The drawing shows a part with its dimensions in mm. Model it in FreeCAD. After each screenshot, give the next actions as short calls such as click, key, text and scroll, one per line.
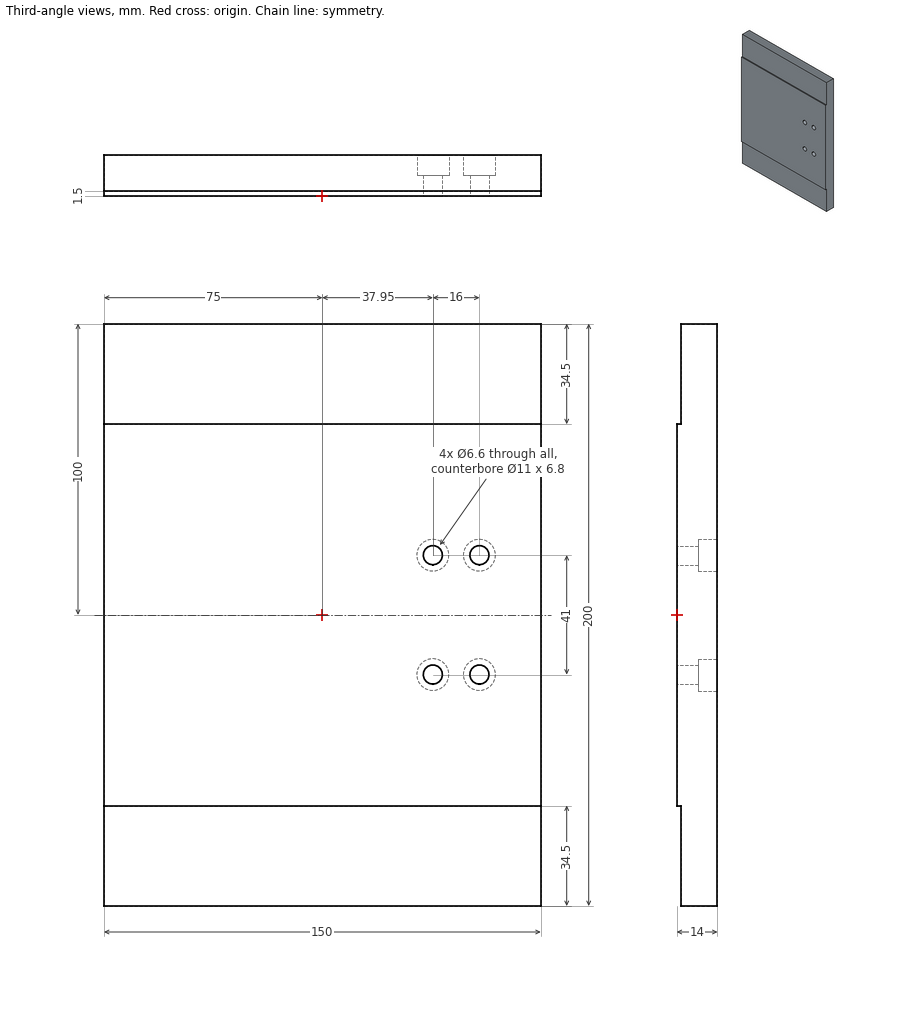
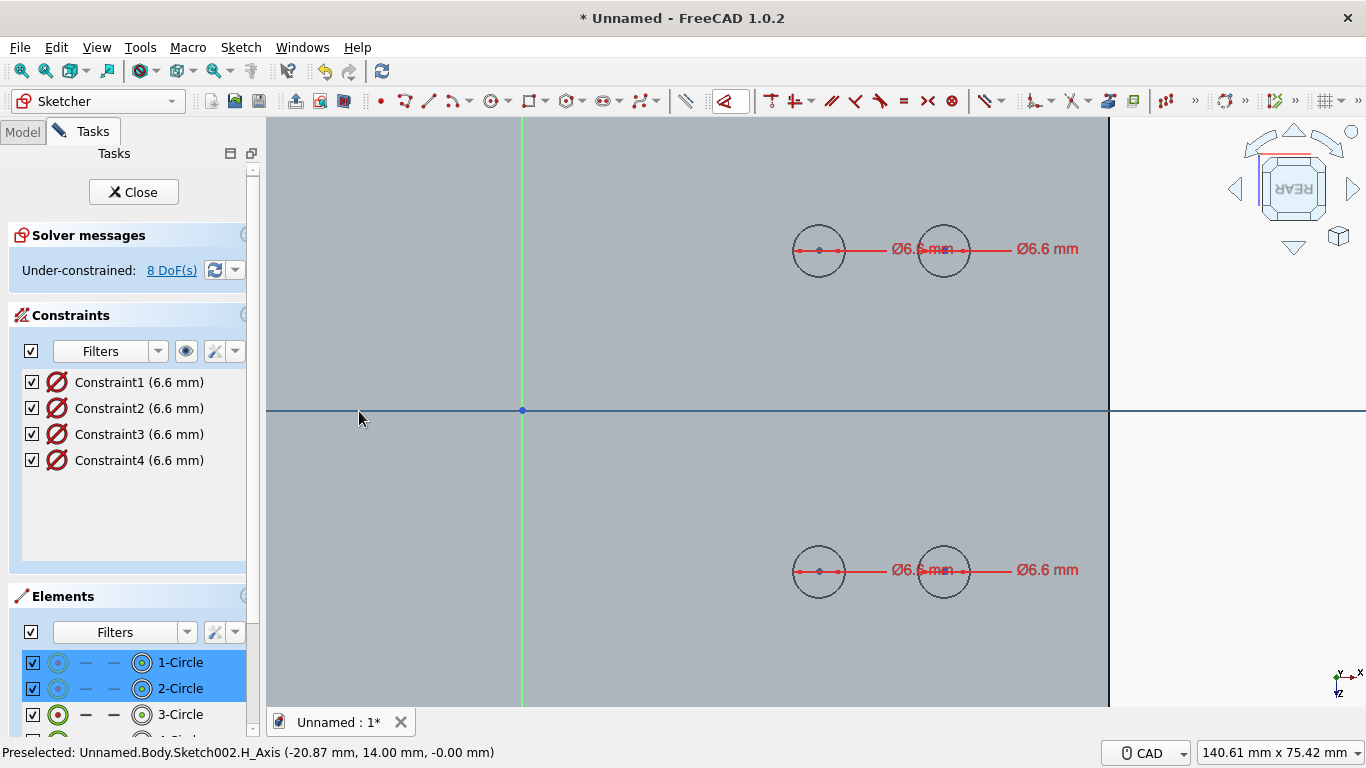
key(s)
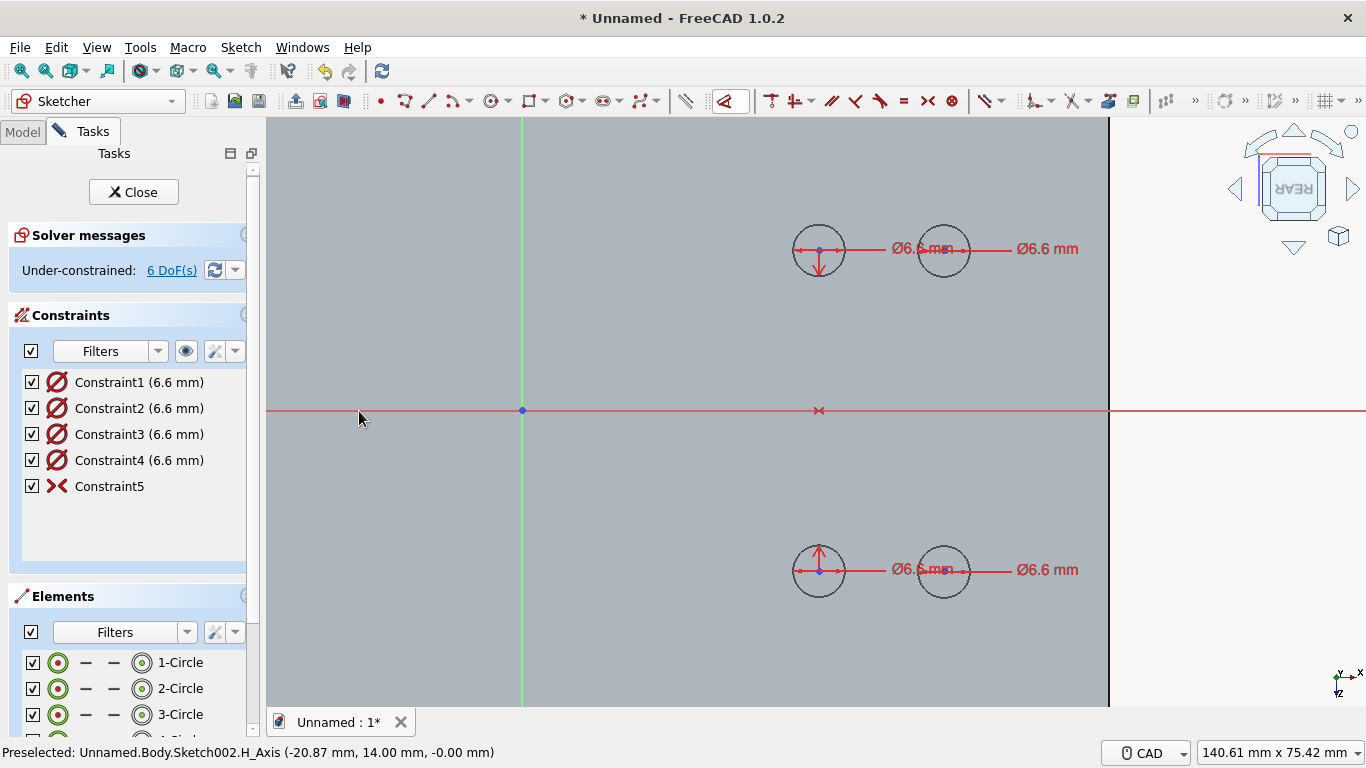
click(944, 572)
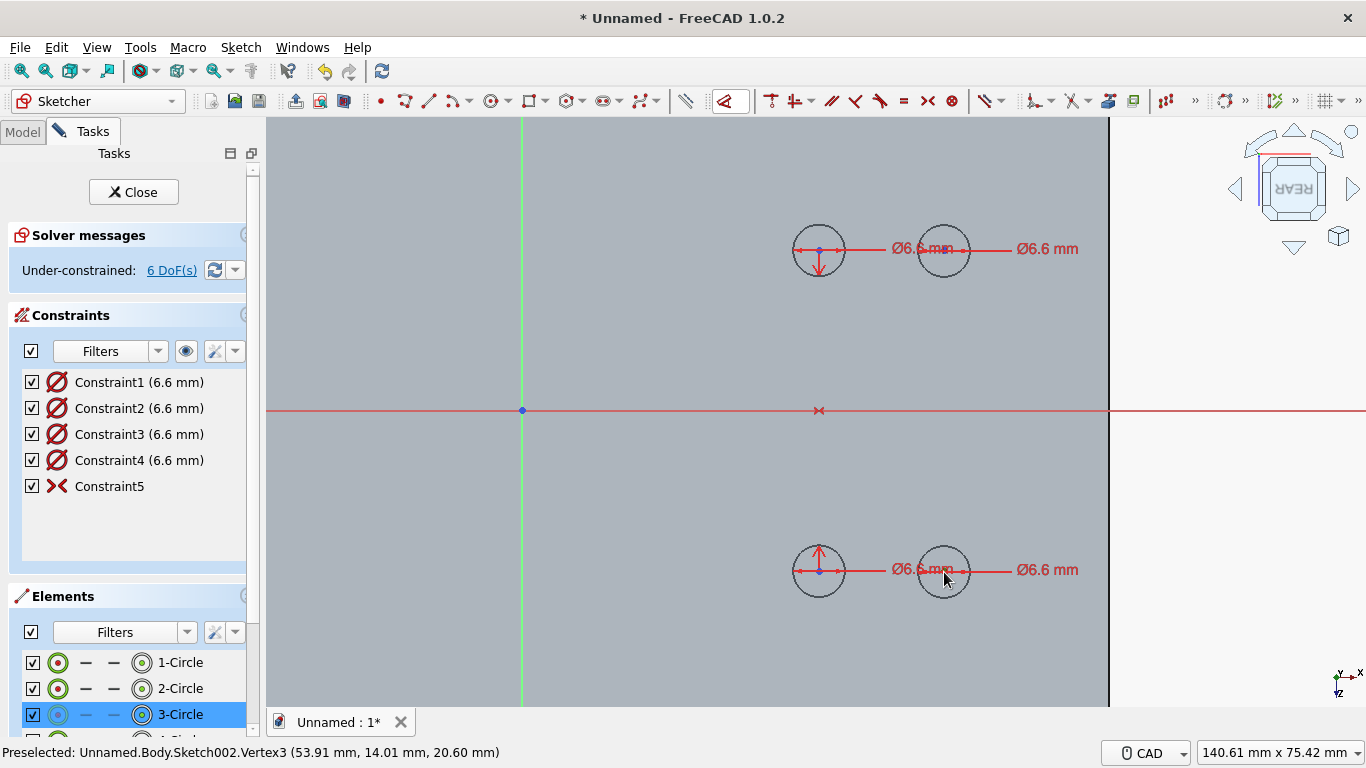
click(944, 251)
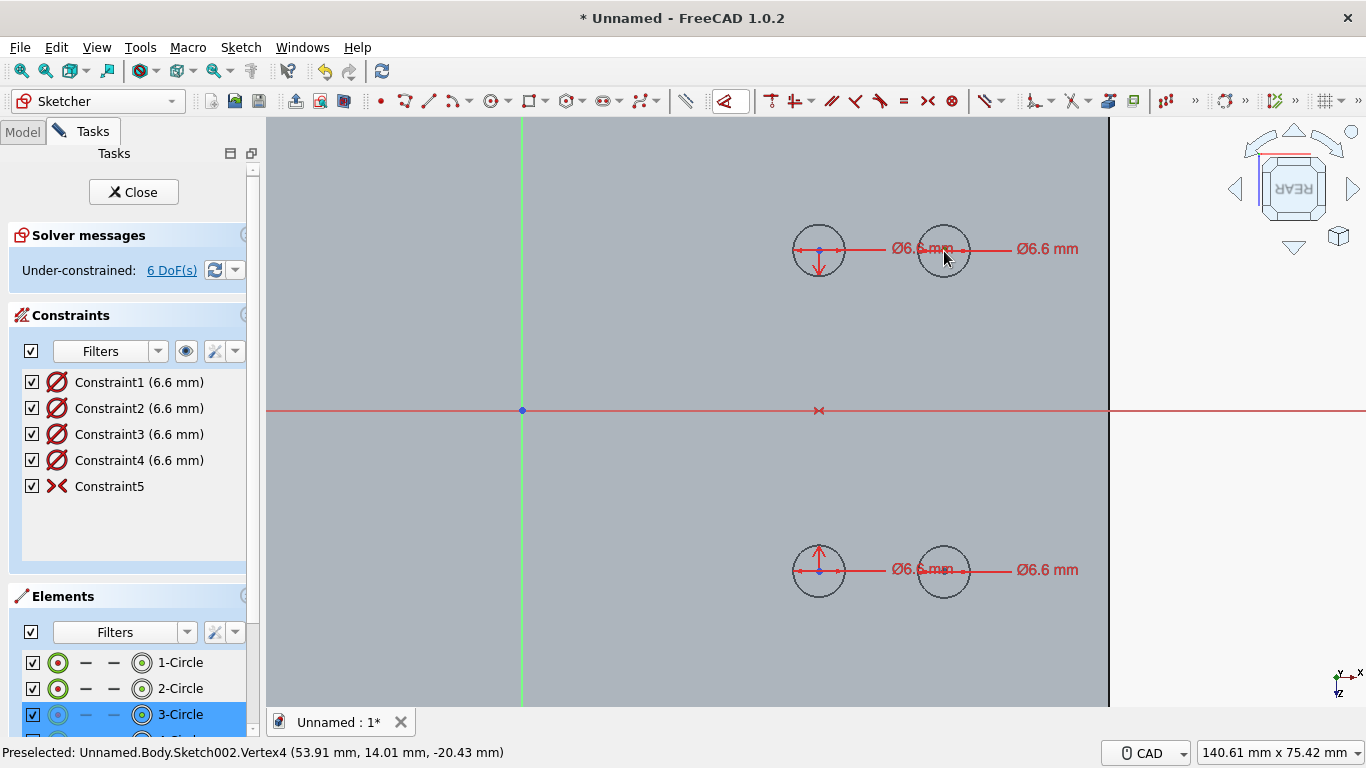
click(359, 411)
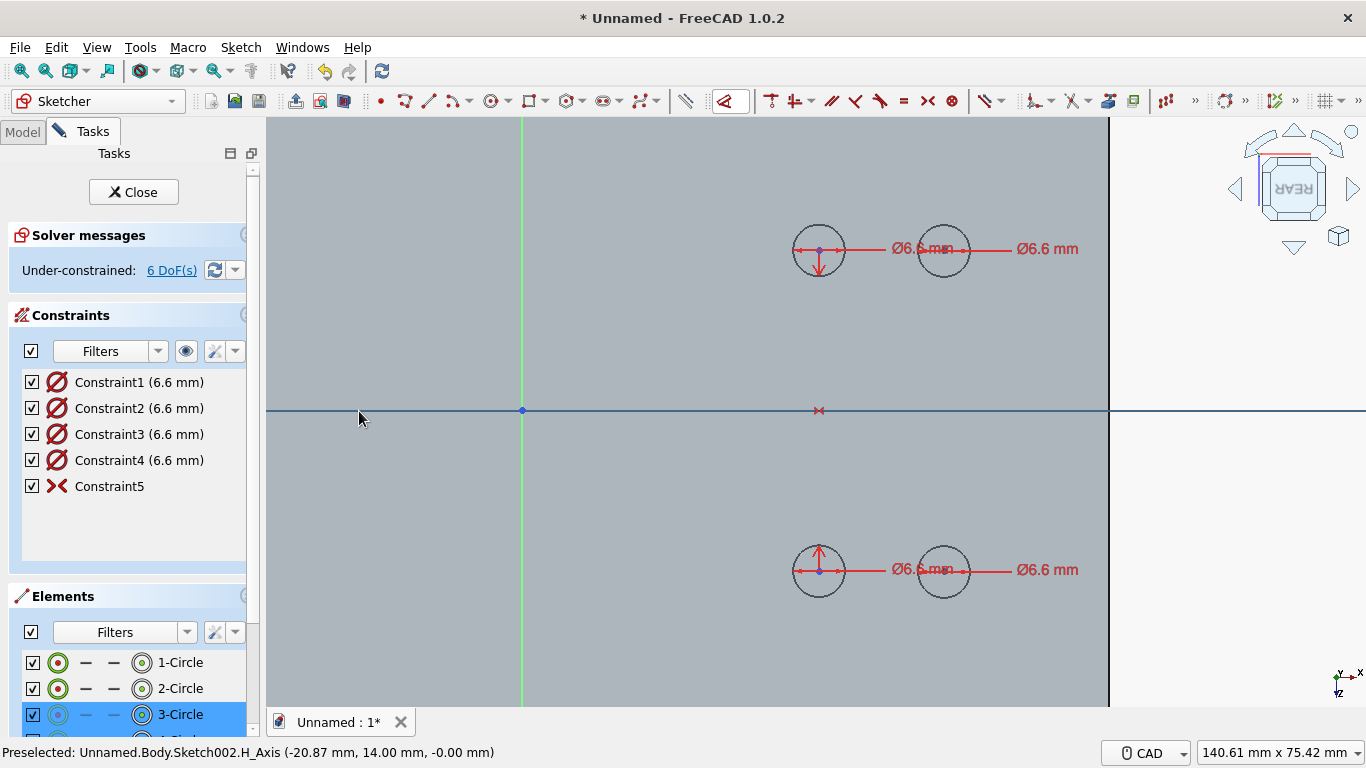
click(928, 102)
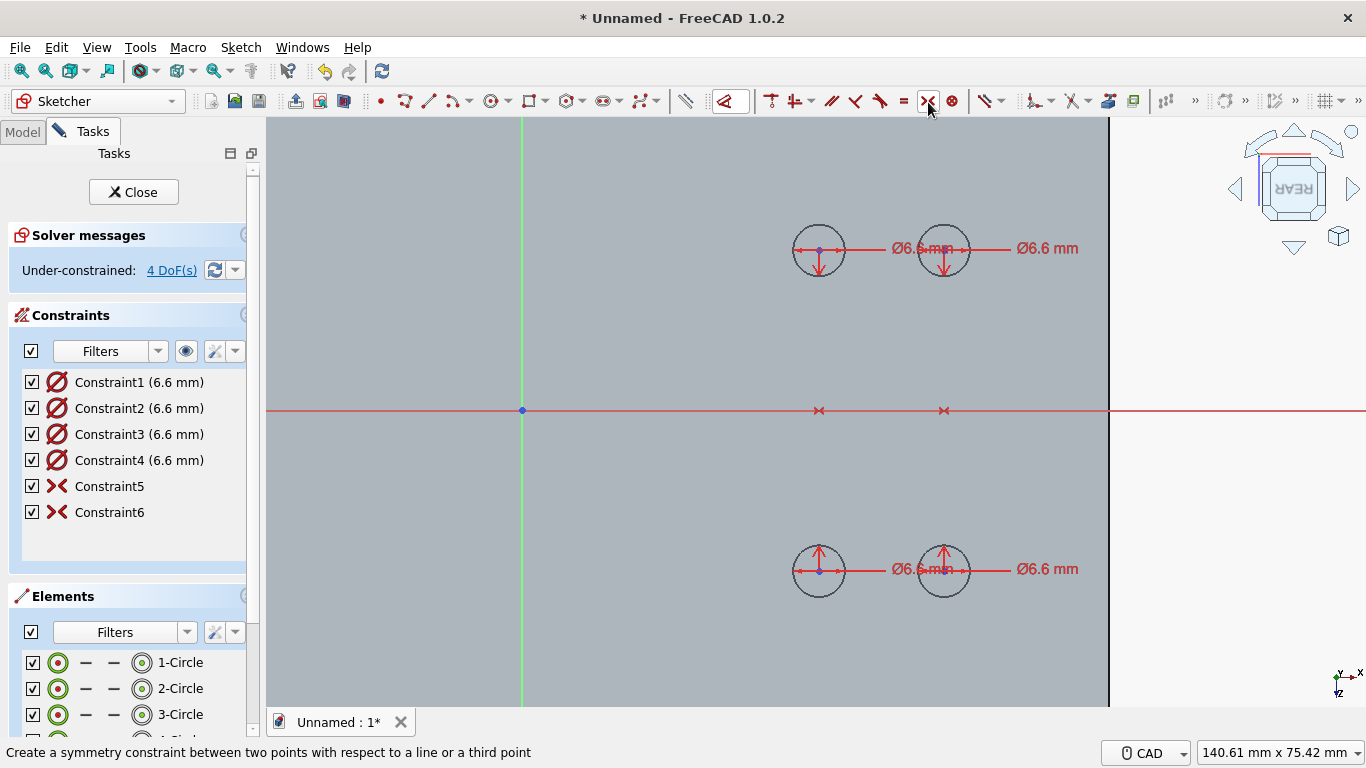
key(d)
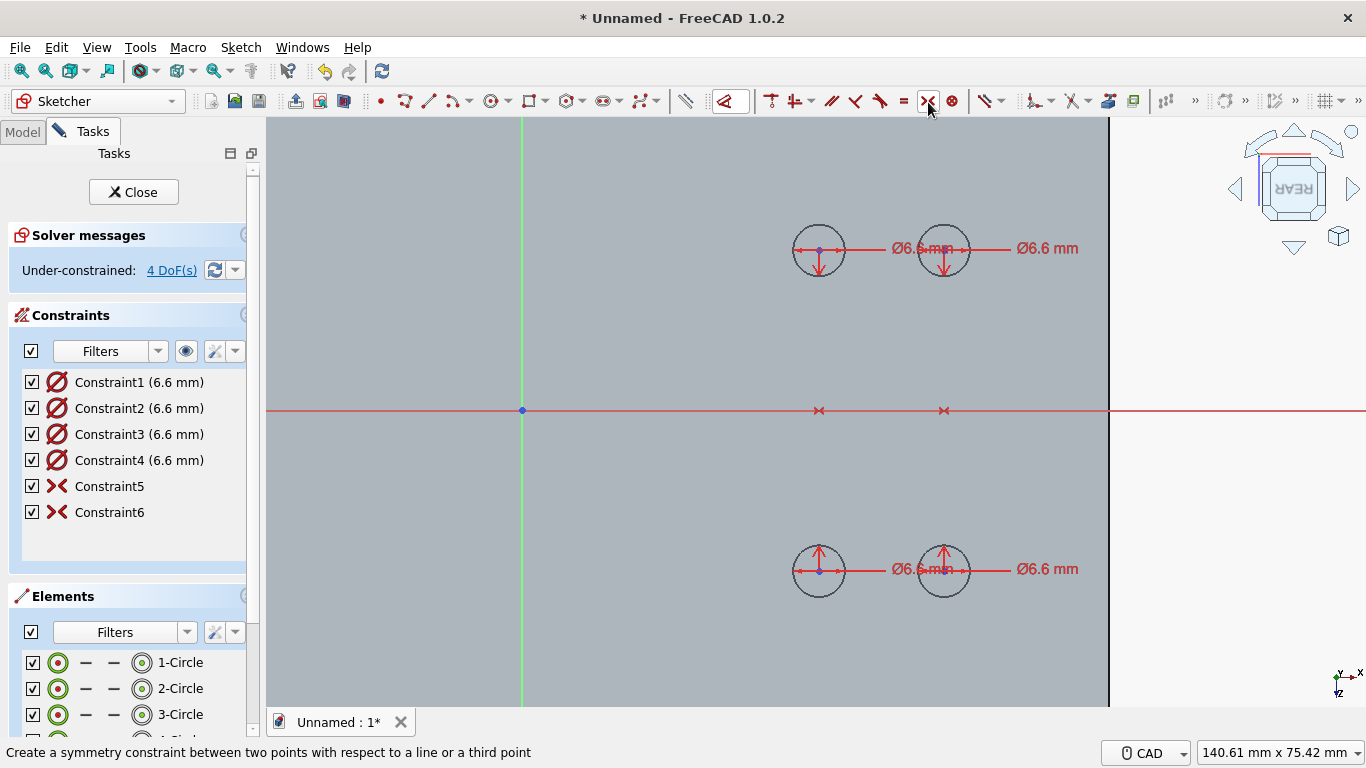
click(819, 571)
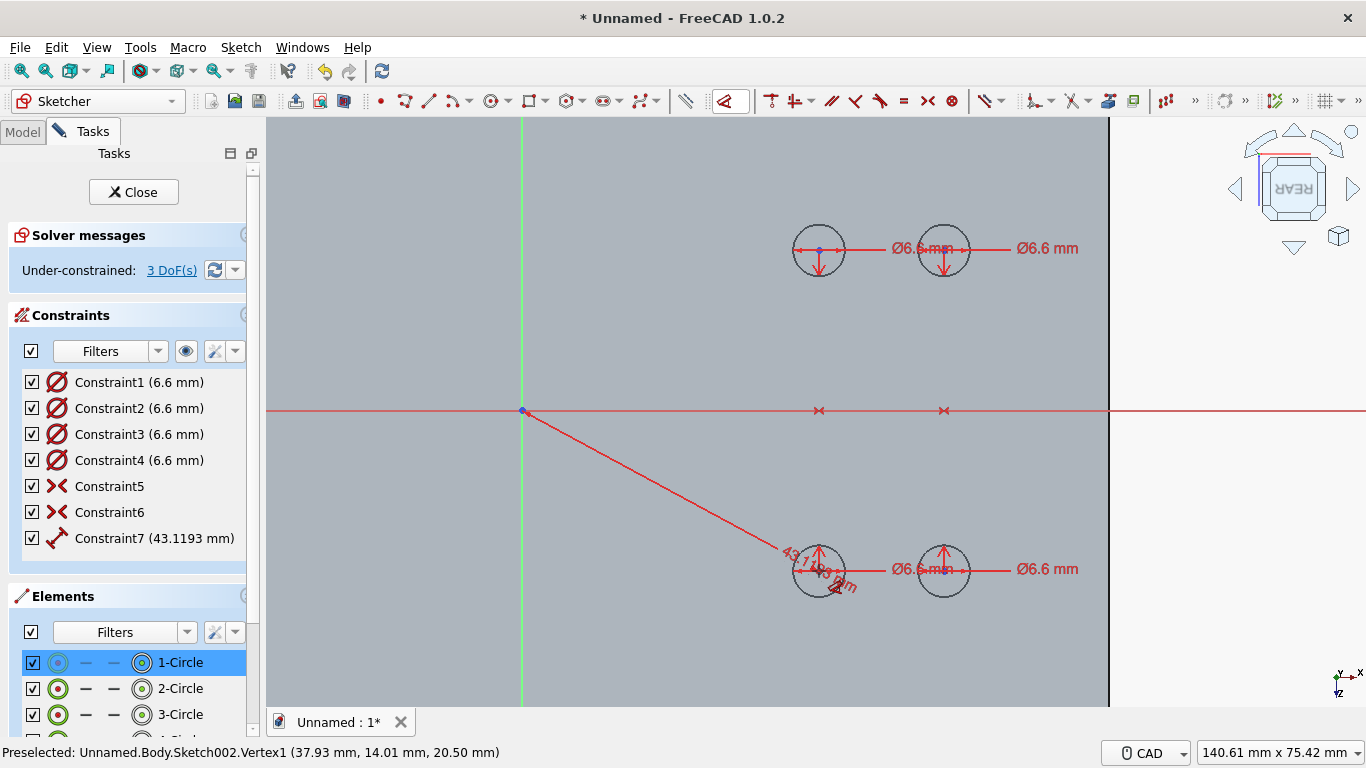
click(819, 250)
click(853, 337)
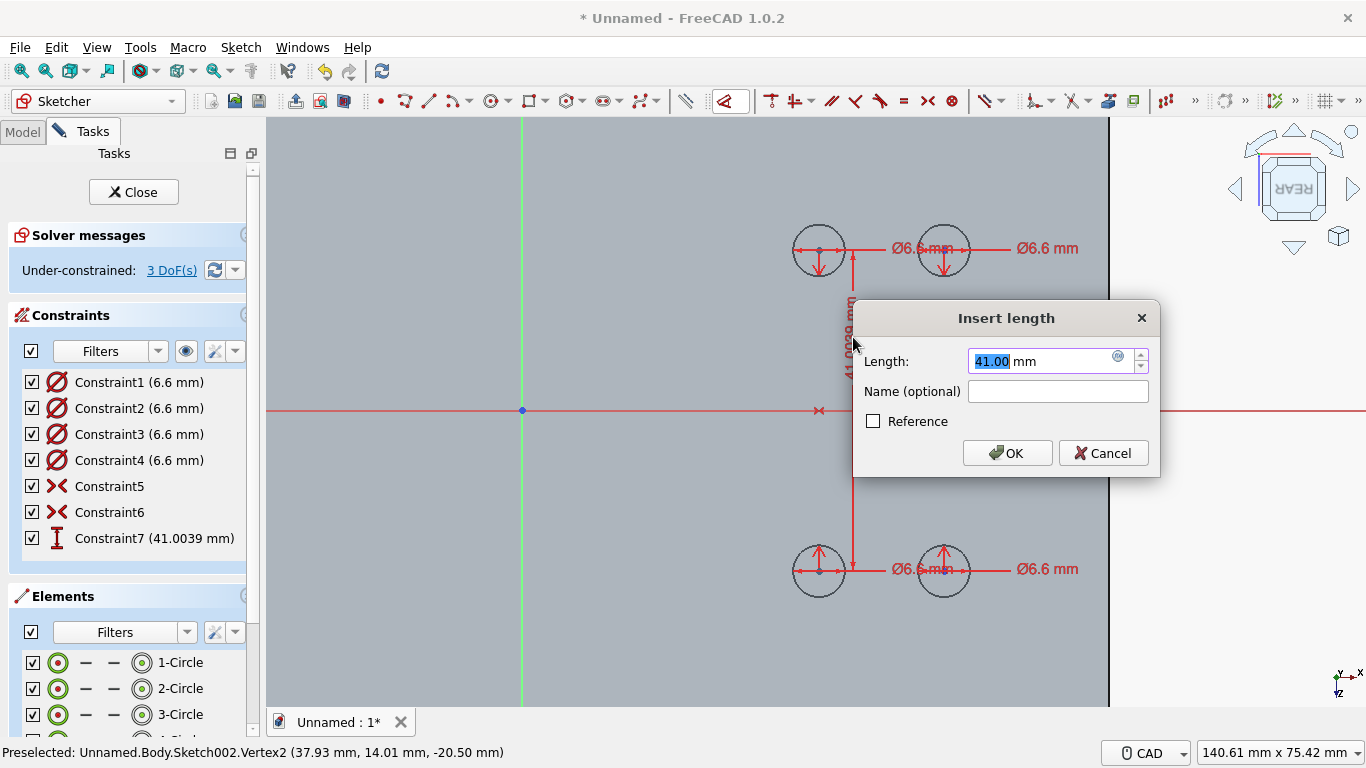
text(41)
key(Return)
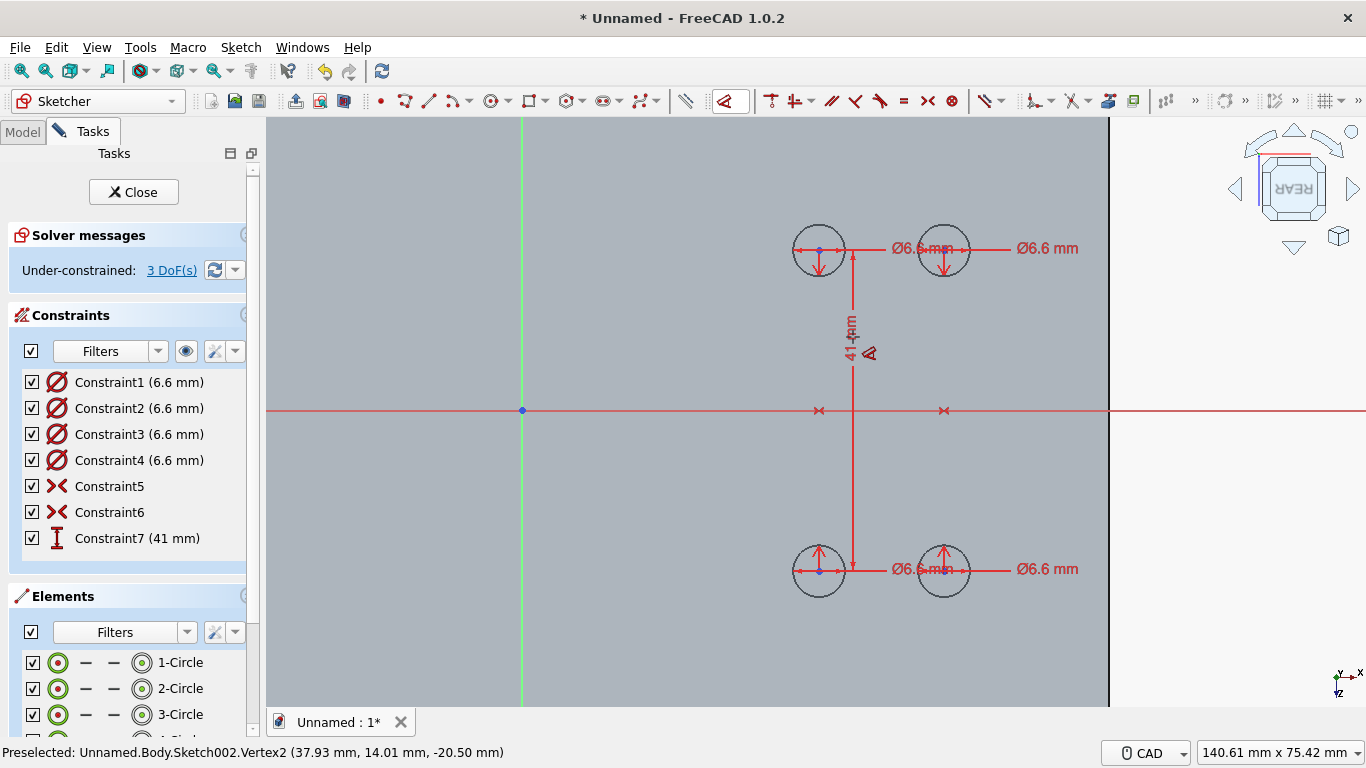
click(819, 571)